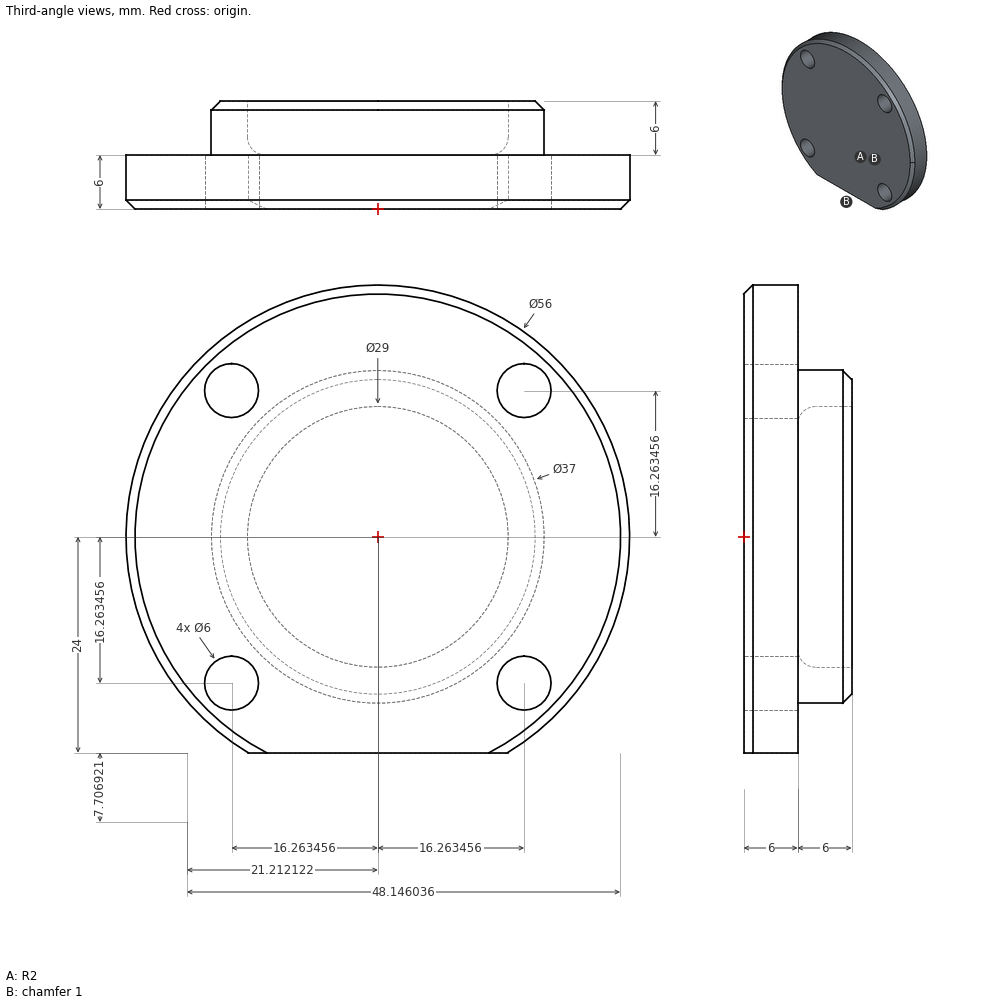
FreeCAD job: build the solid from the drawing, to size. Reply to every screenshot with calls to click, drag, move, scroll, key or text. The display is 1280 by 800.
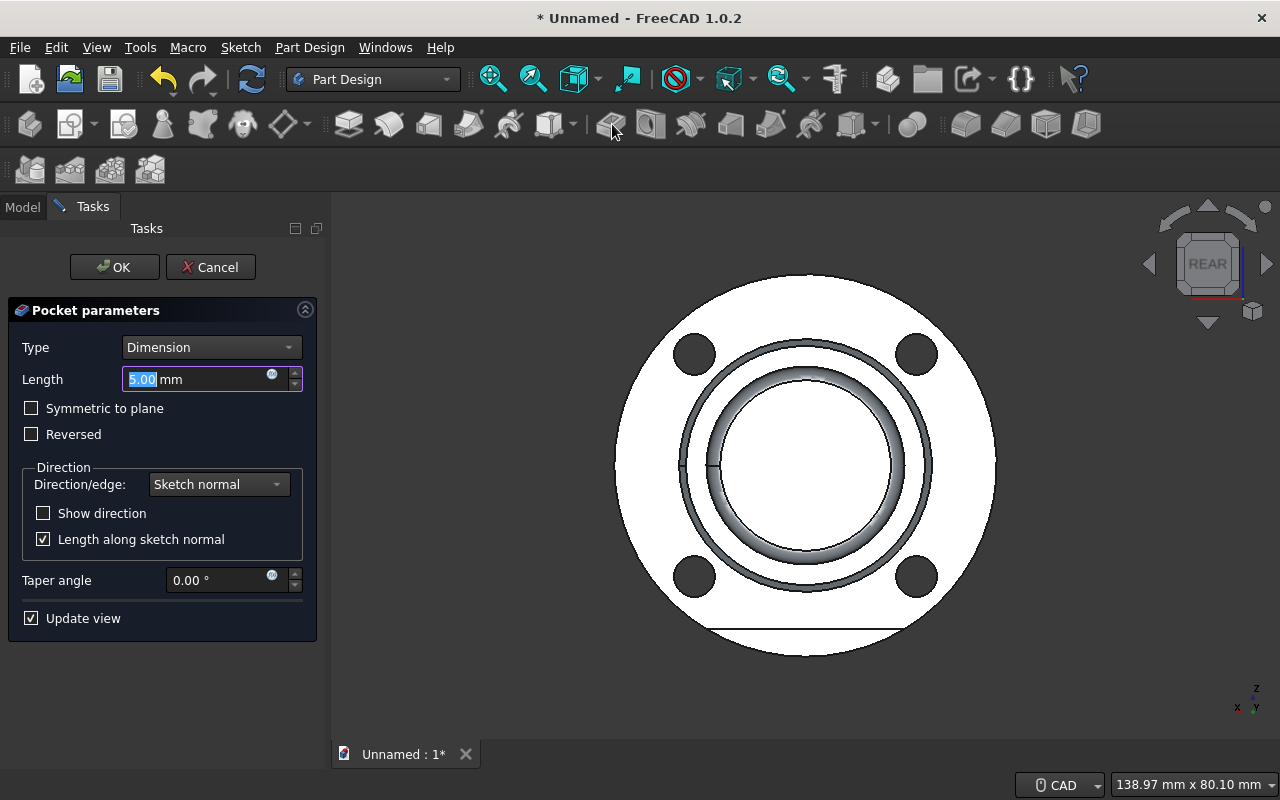
text(6)
key(Tab)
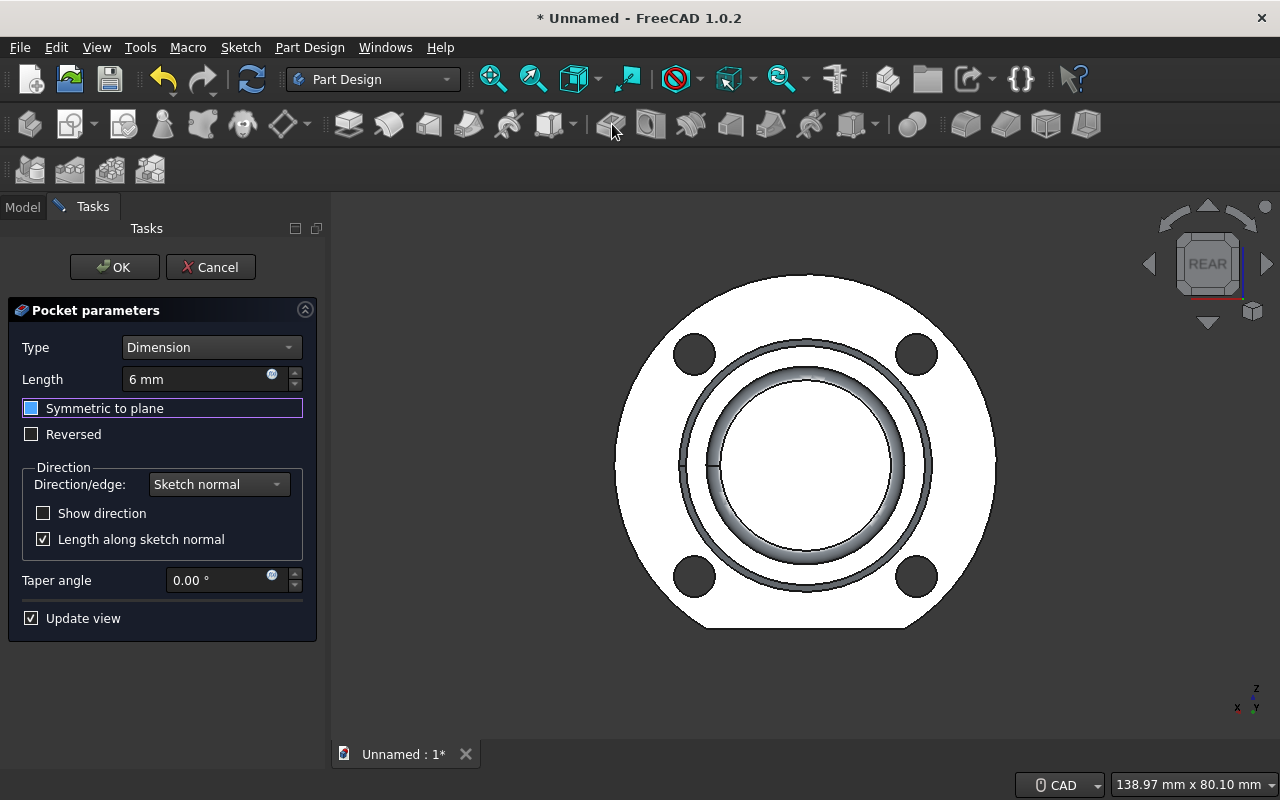
click(115, 267)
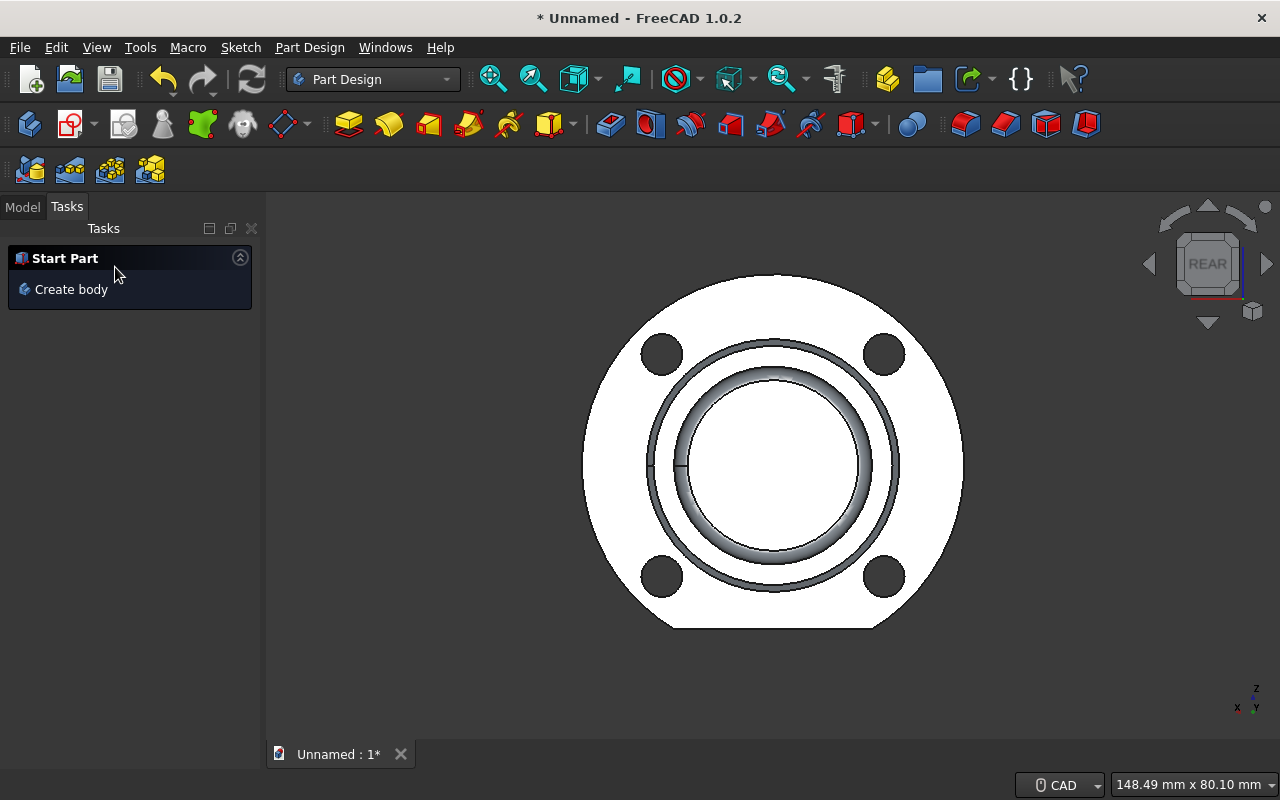
key(0)